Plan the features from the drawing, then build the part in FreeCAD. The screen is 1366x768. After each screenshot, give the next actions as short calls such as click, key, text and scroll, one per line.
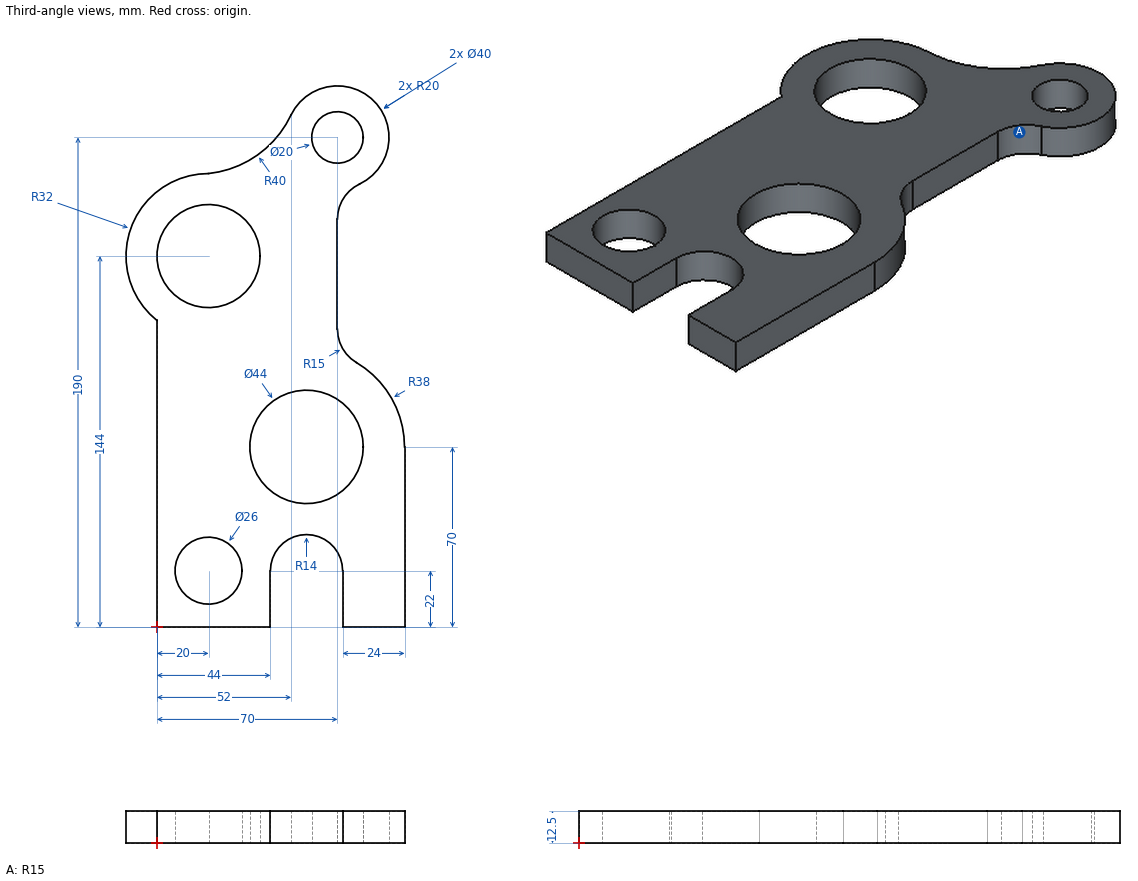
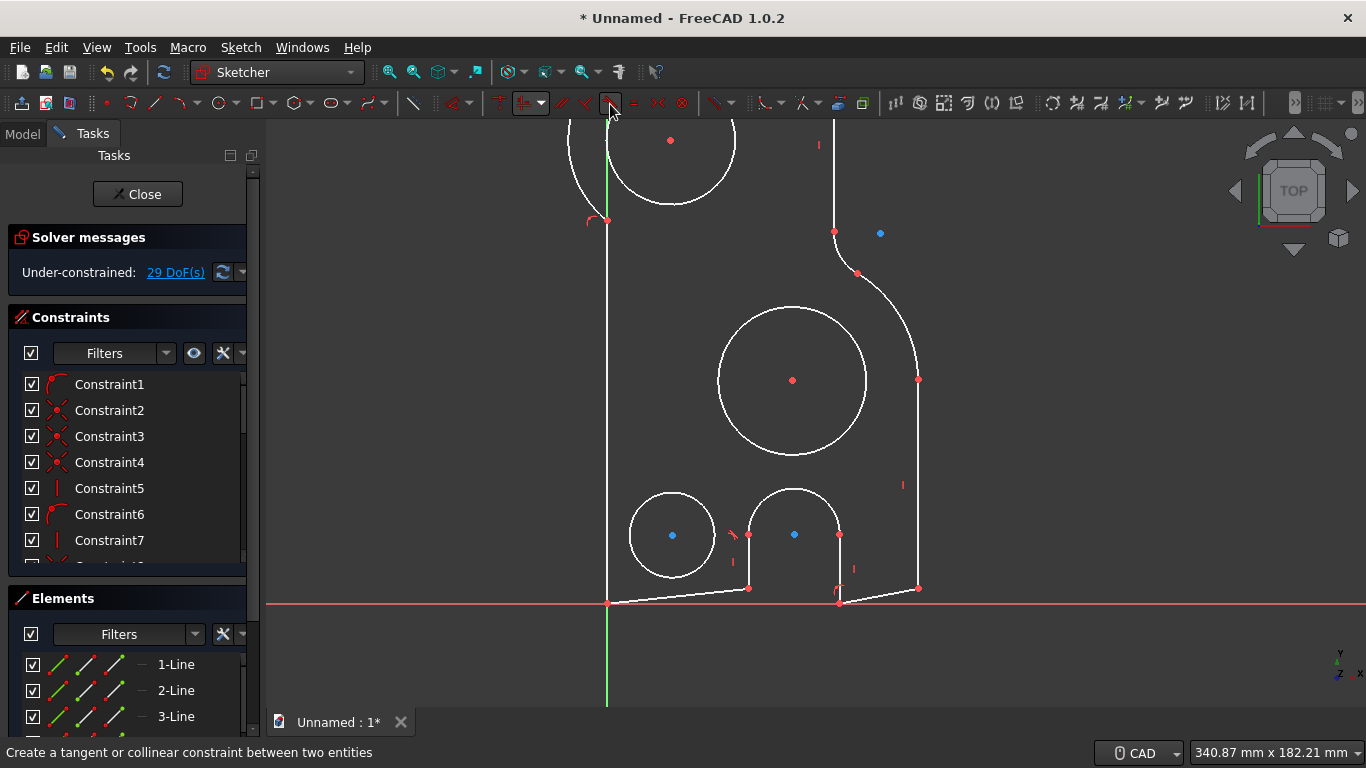
click(840, 555)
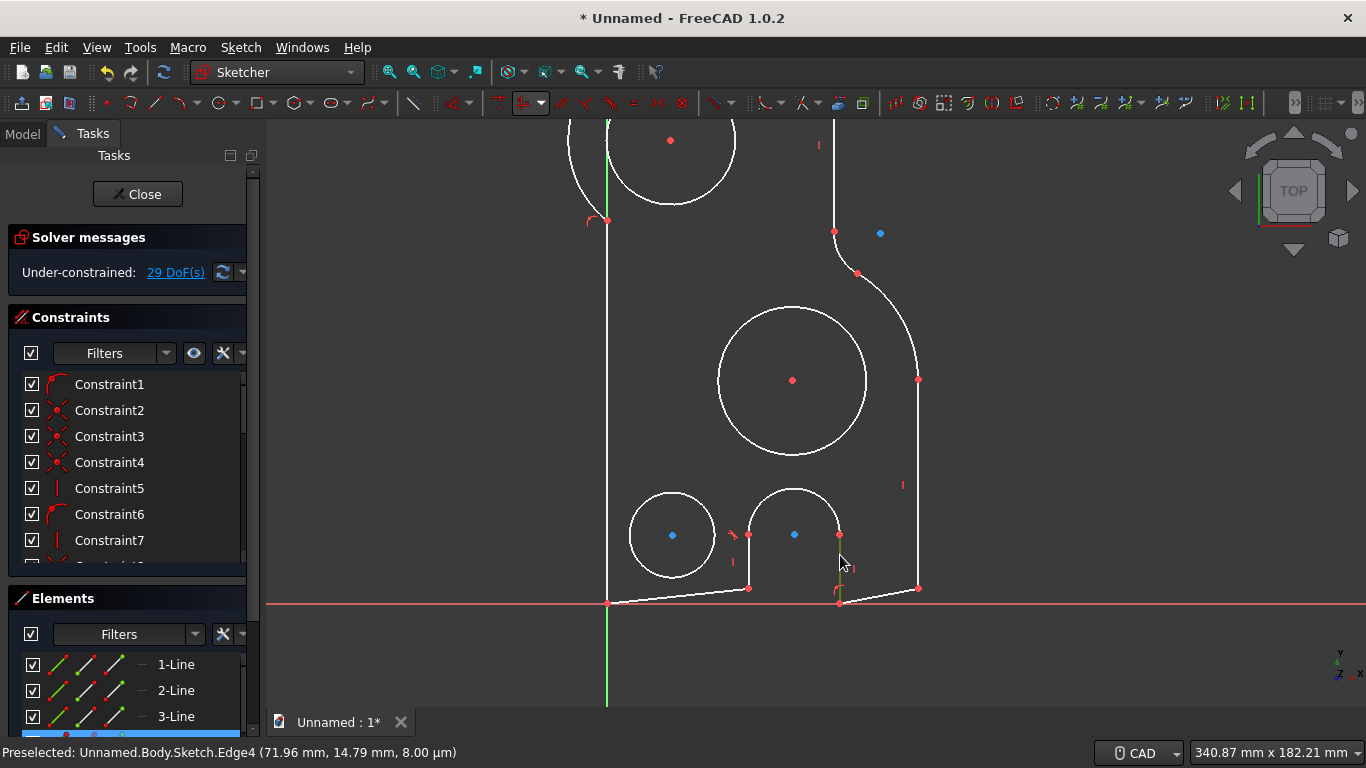
click(821, 497)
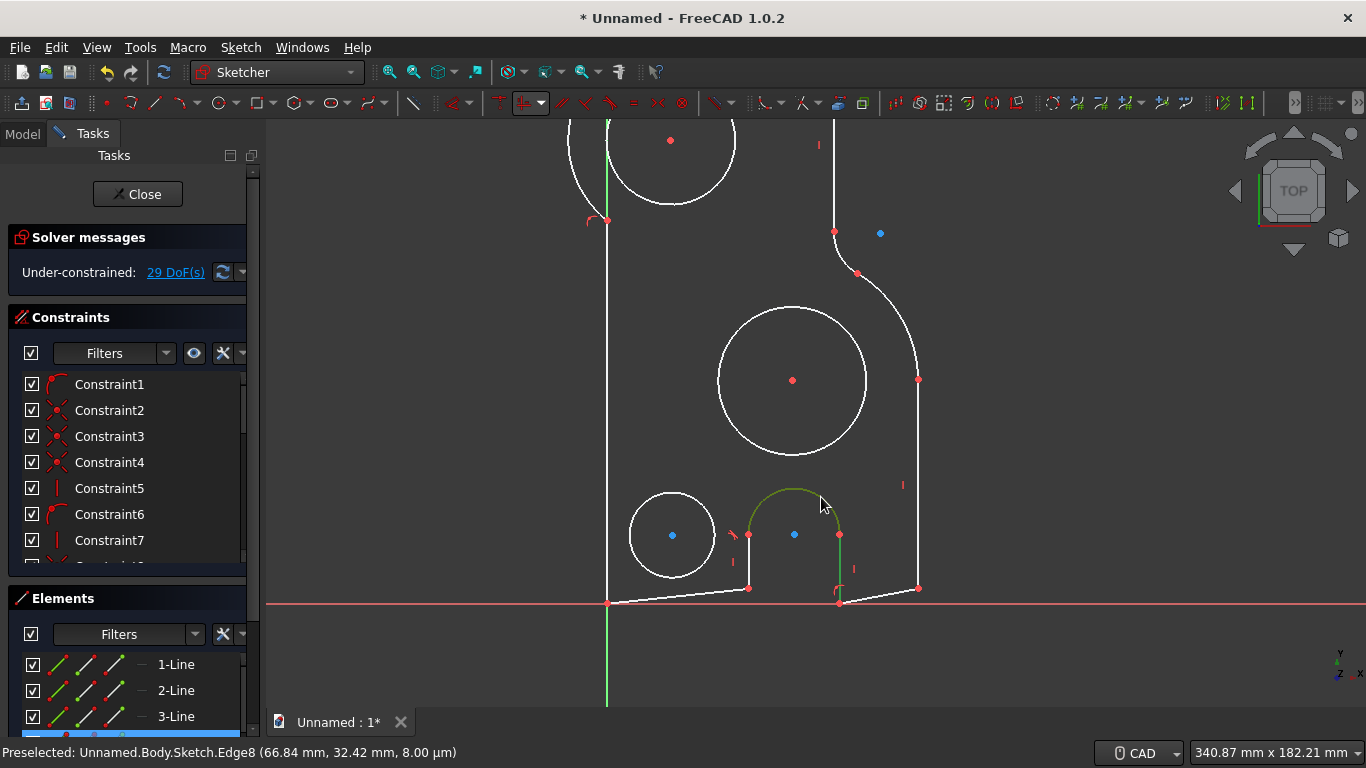
click(610, 104)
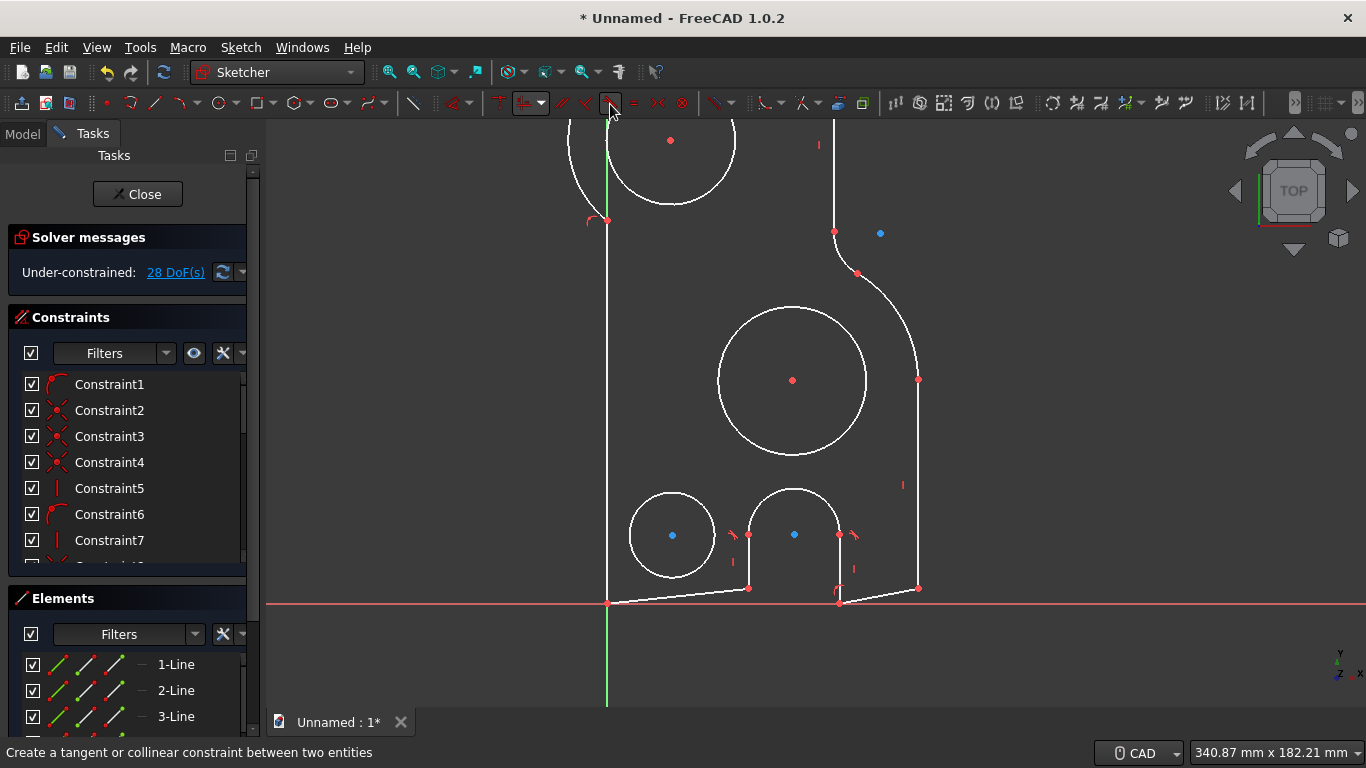
click(918, 526)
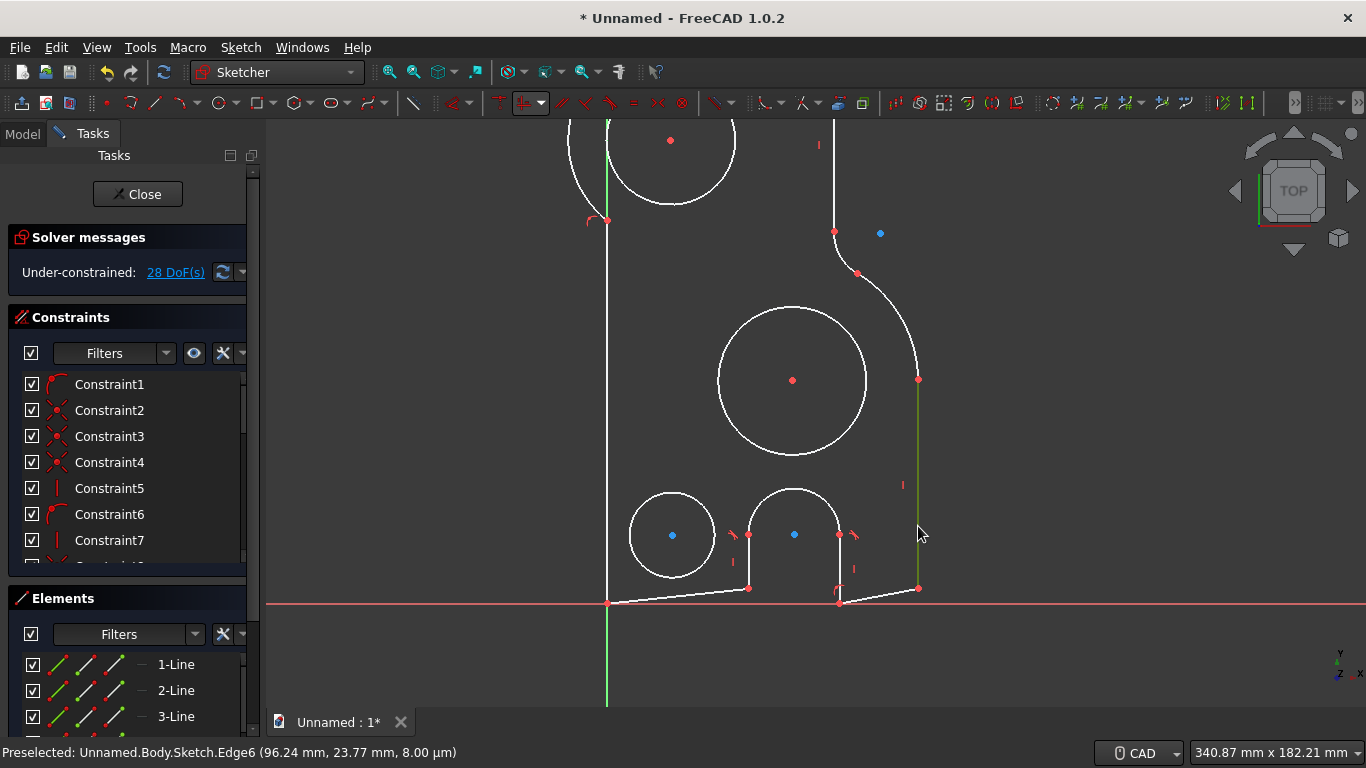
click(912, 342)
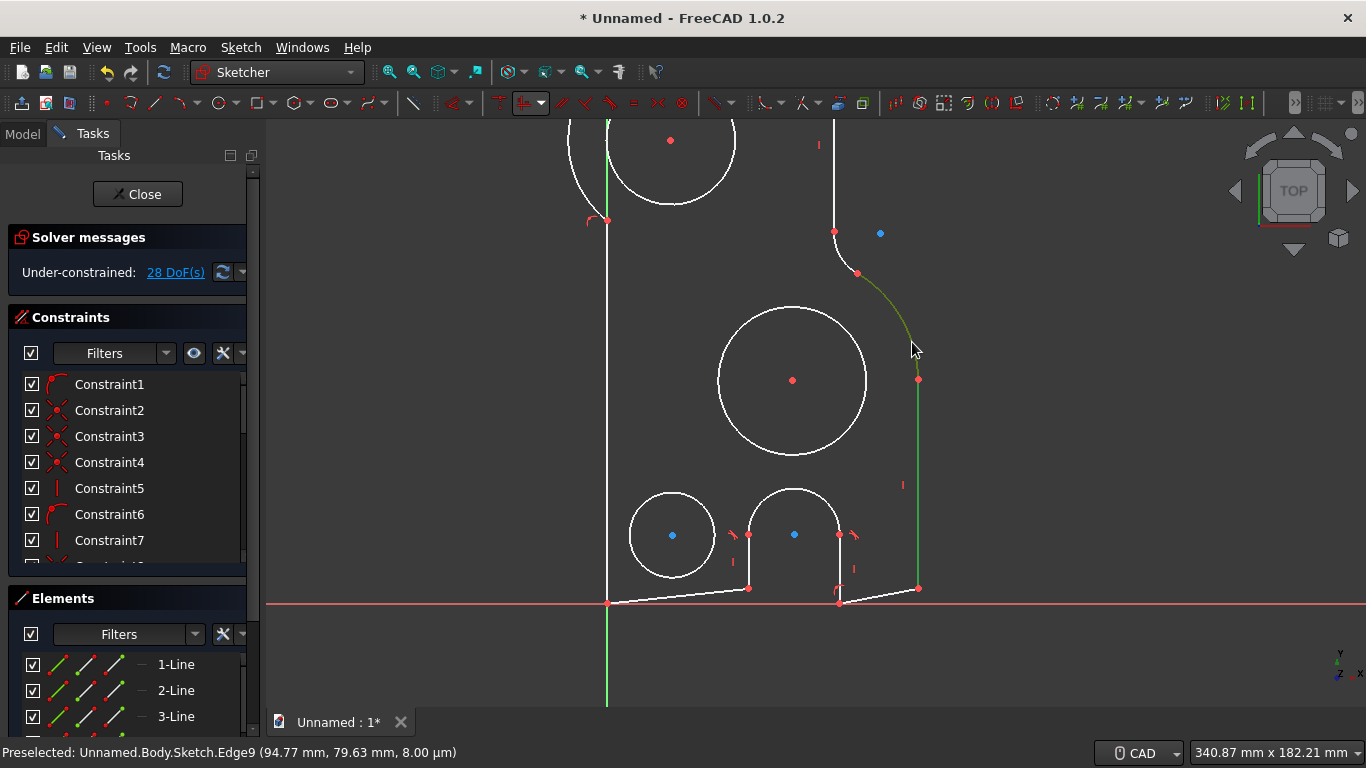
click(610, 104)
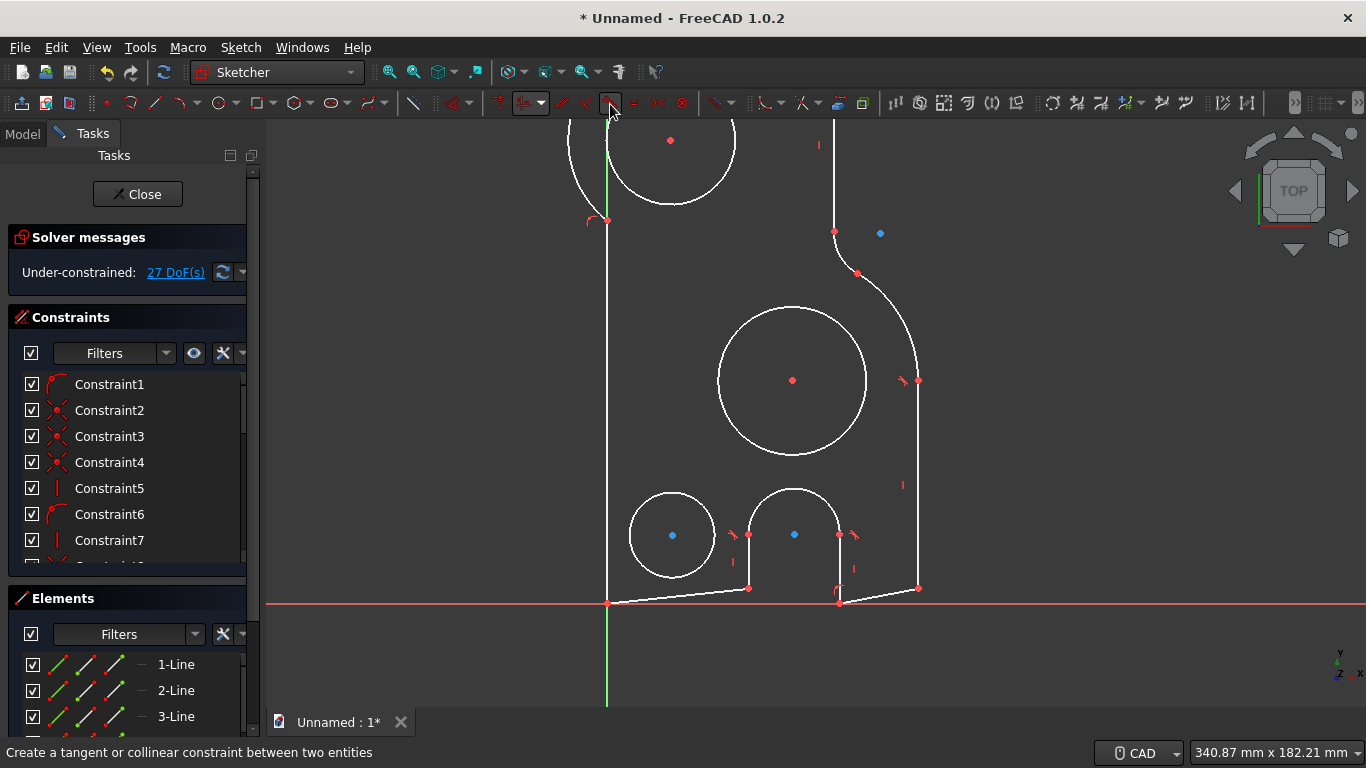
click(834, 179)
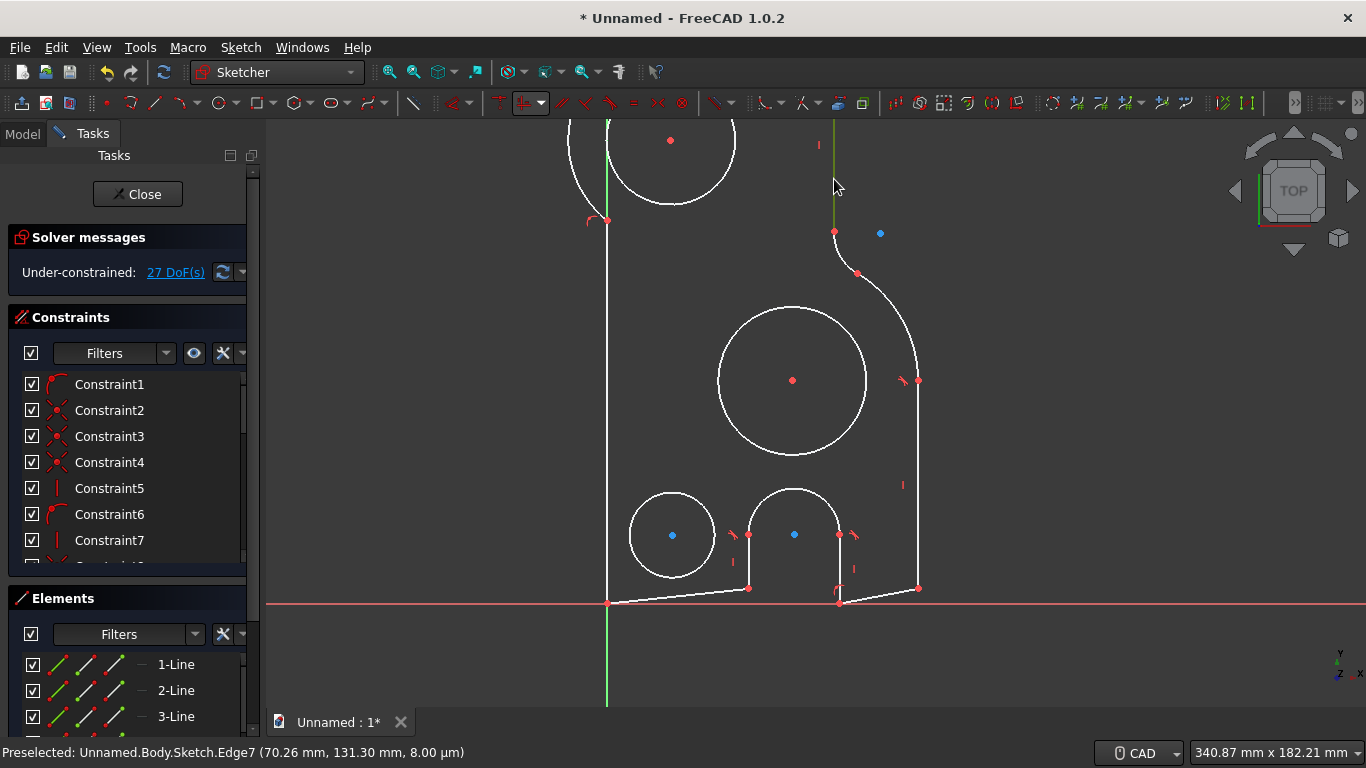
click(836, 247)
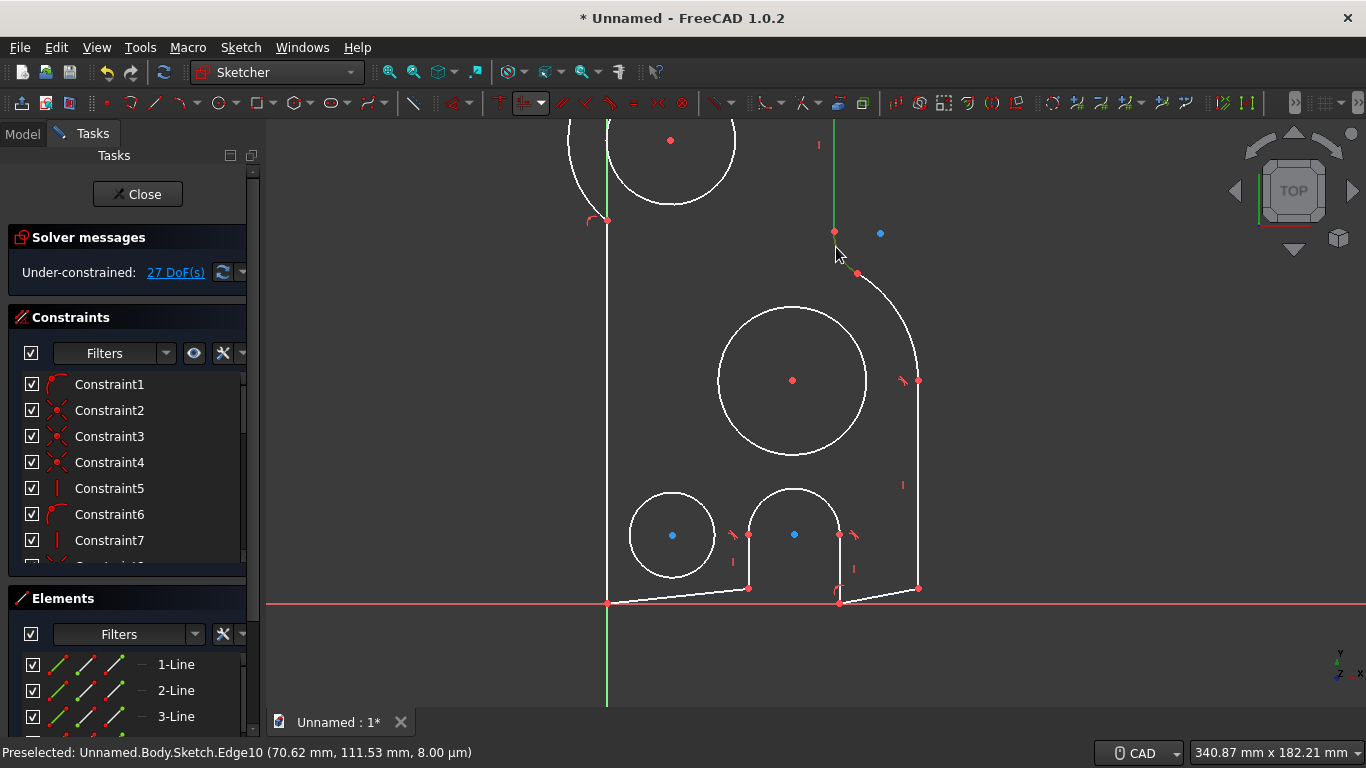
click(610, 104)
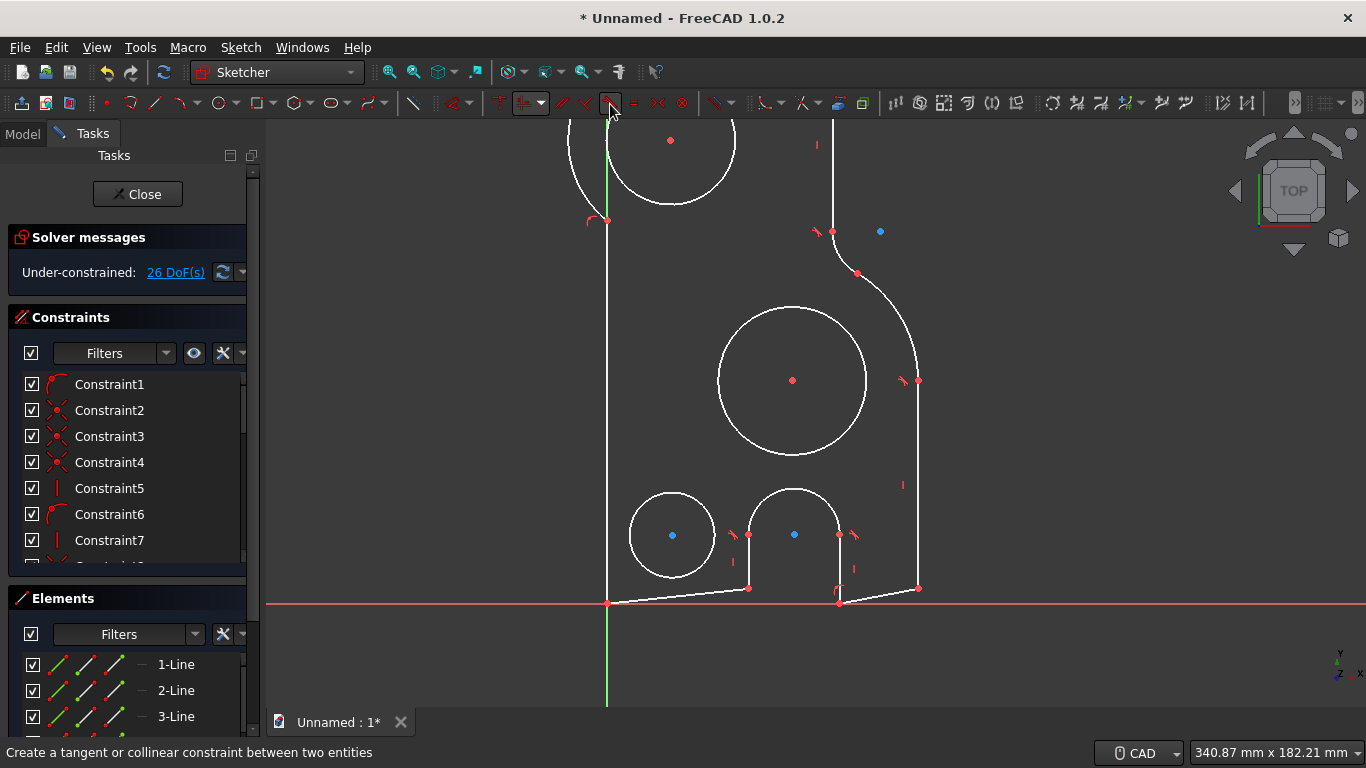
click(912, 343)